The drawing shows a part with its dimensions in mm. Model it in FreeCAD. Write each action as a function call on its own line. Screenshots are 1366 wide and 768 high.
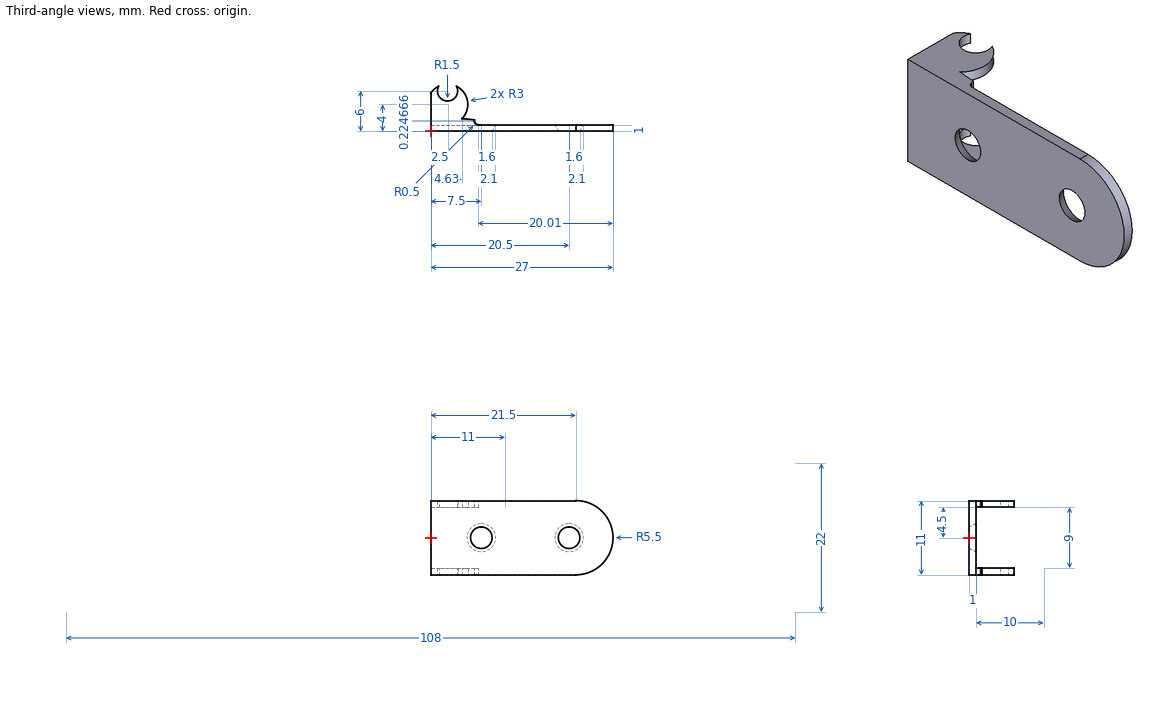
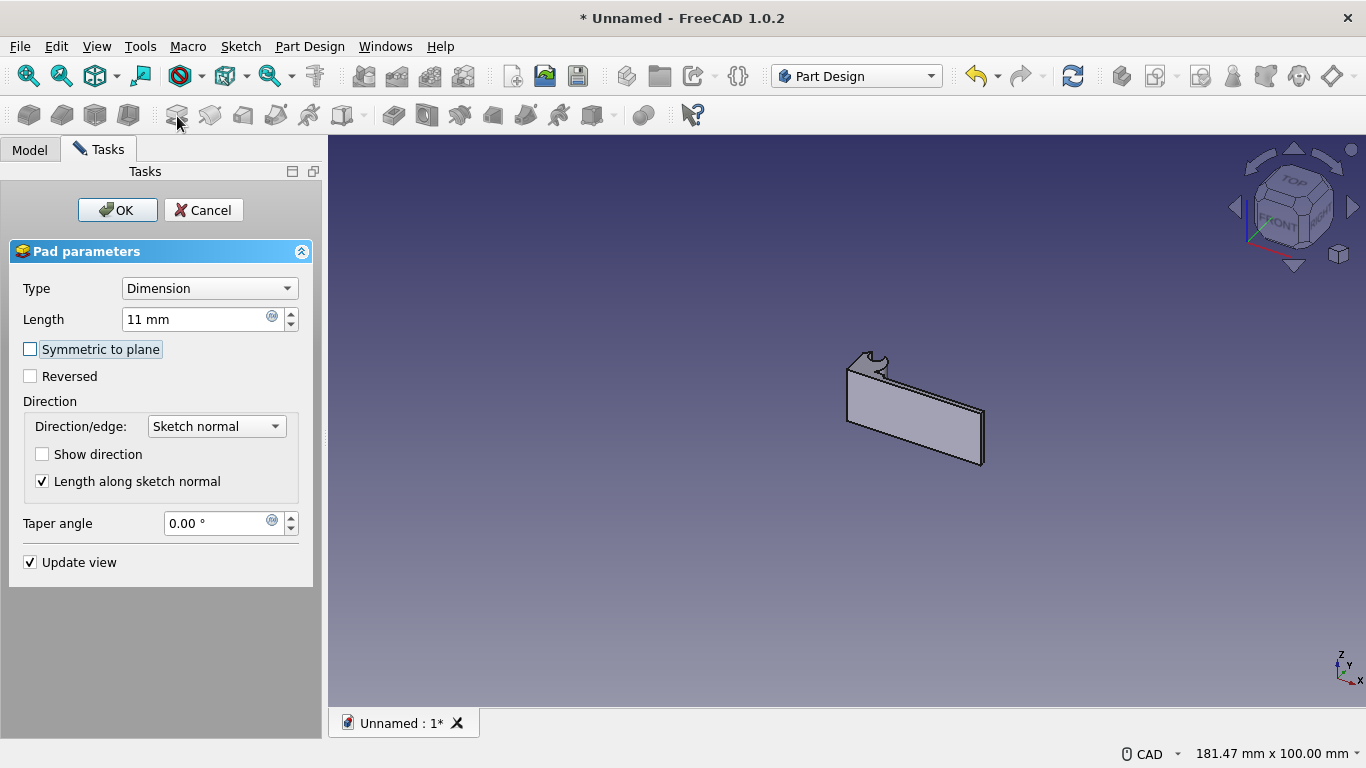
click(31, 349)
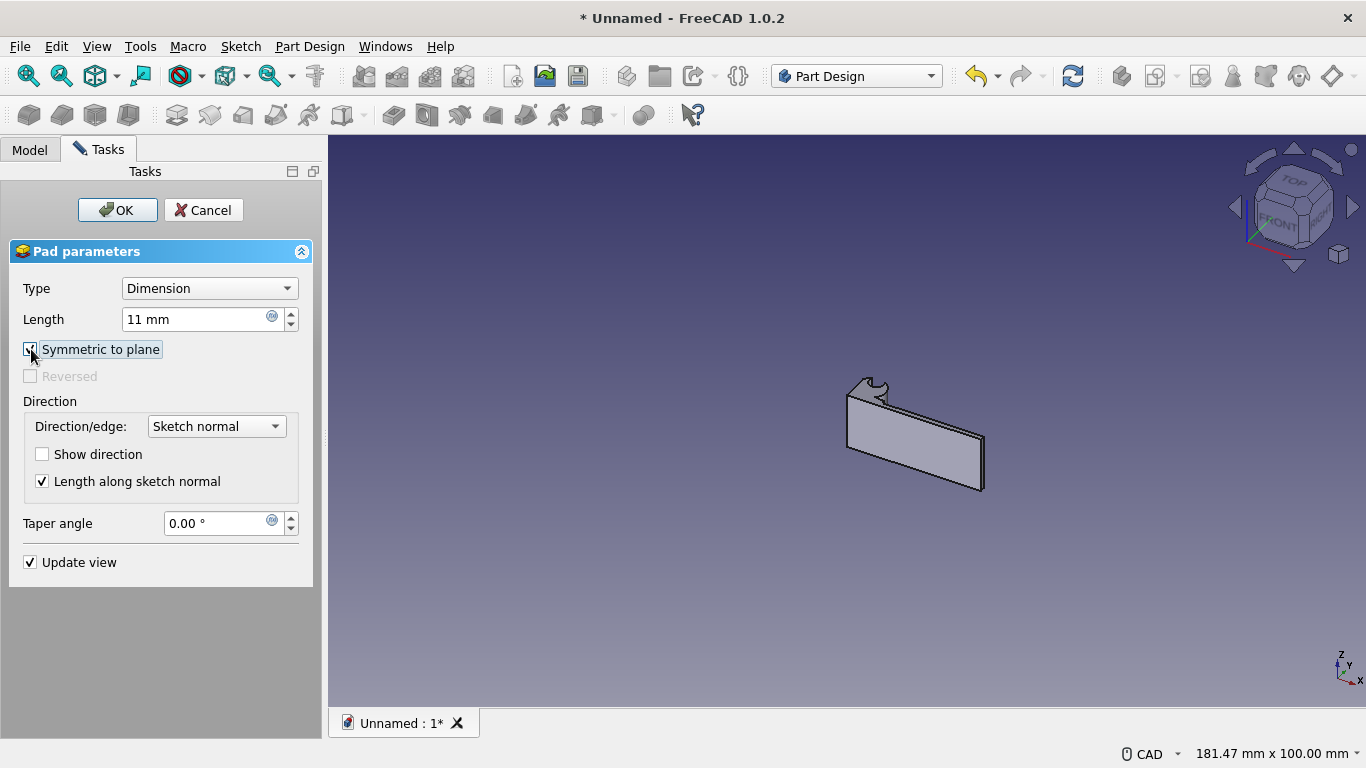
click(118, 210)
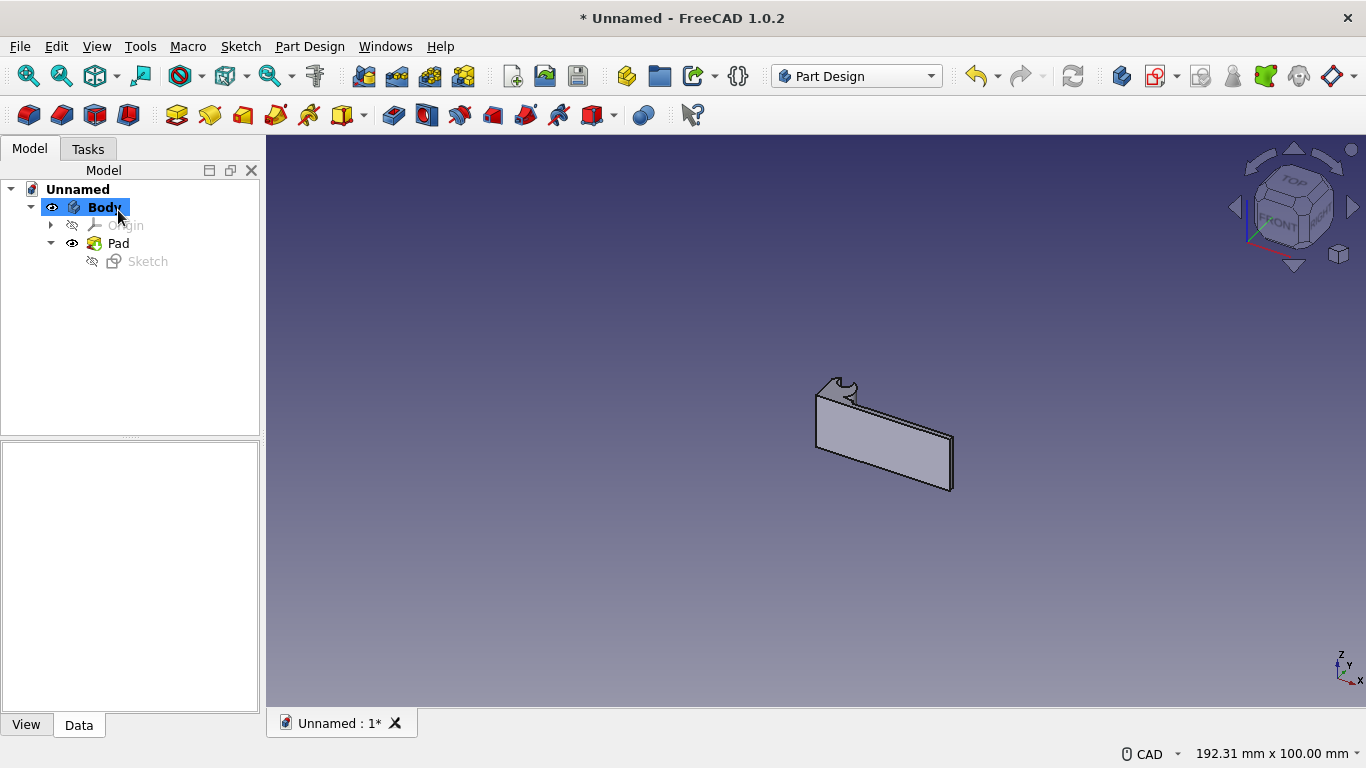
key(v)
key(f)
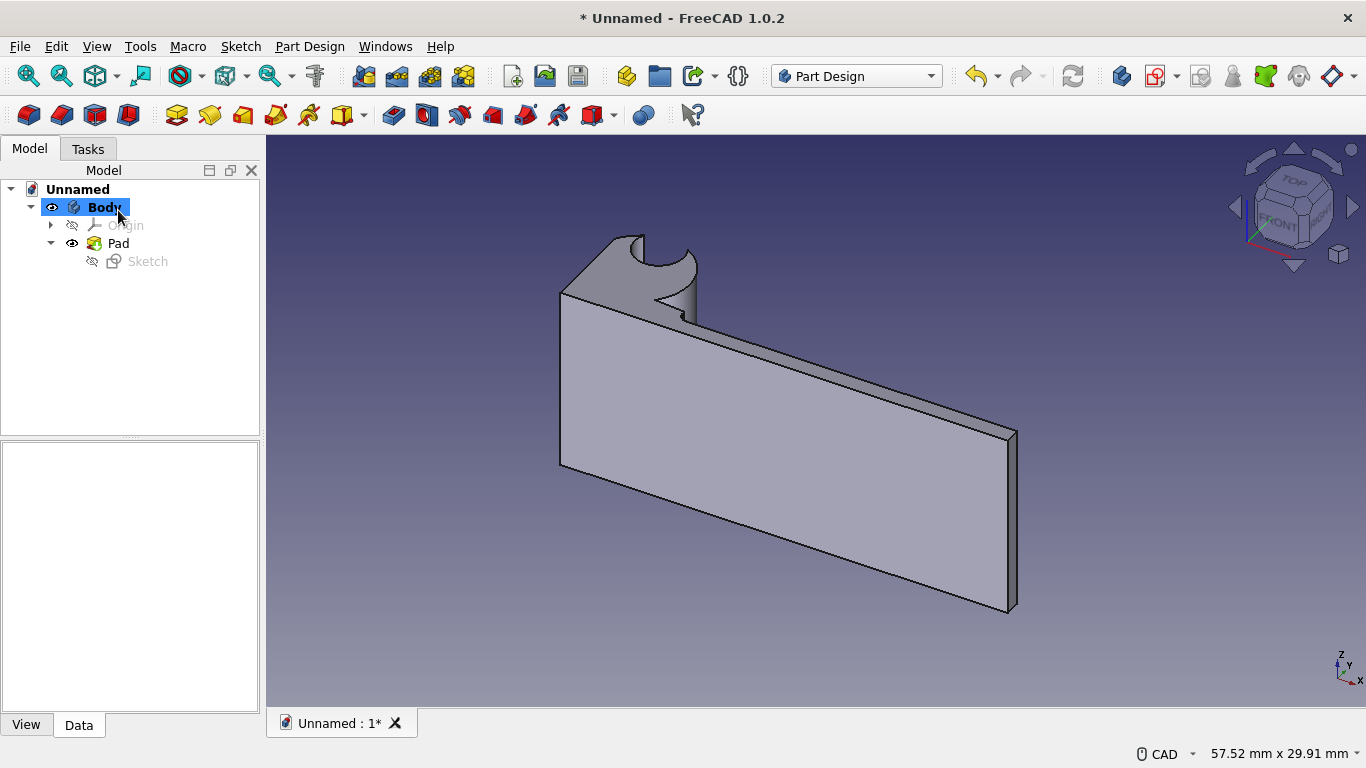
click(1154, 76)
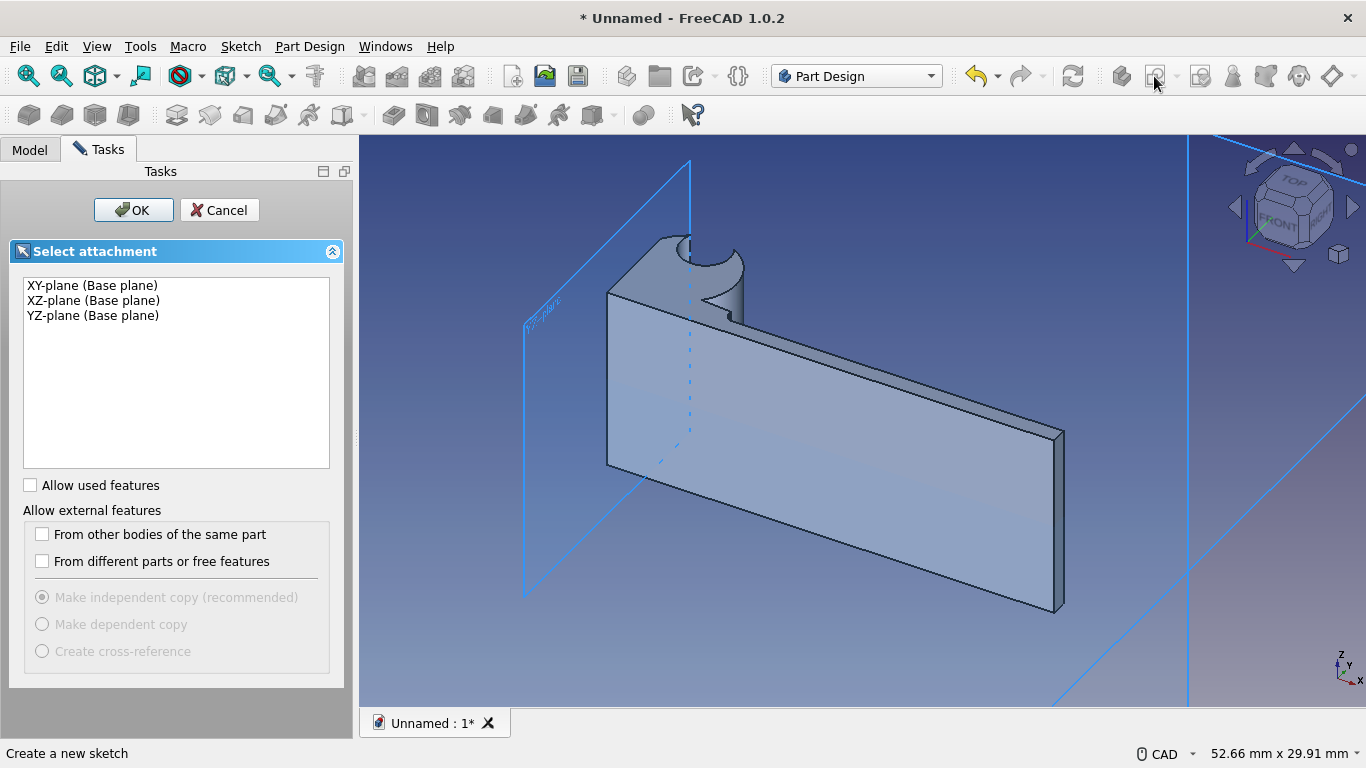
click(84, 300)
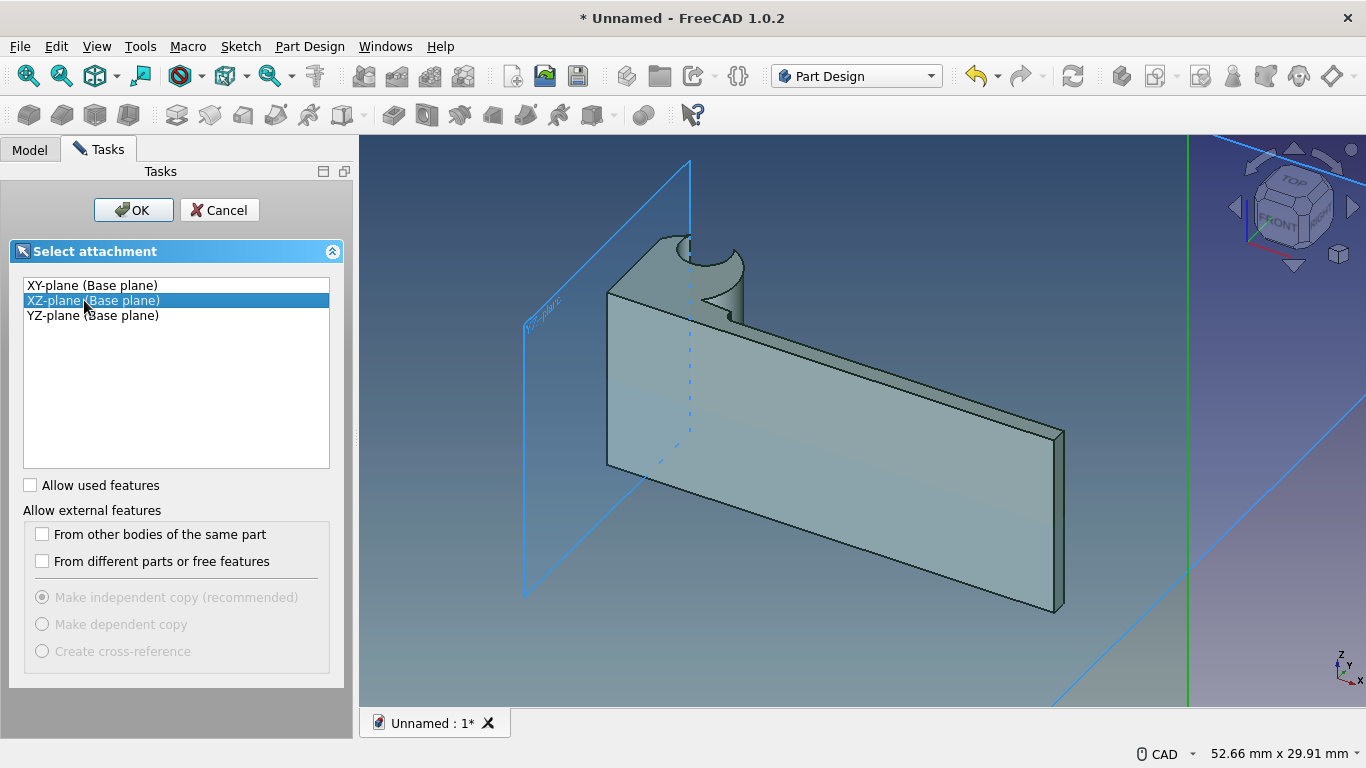
click(134, 210)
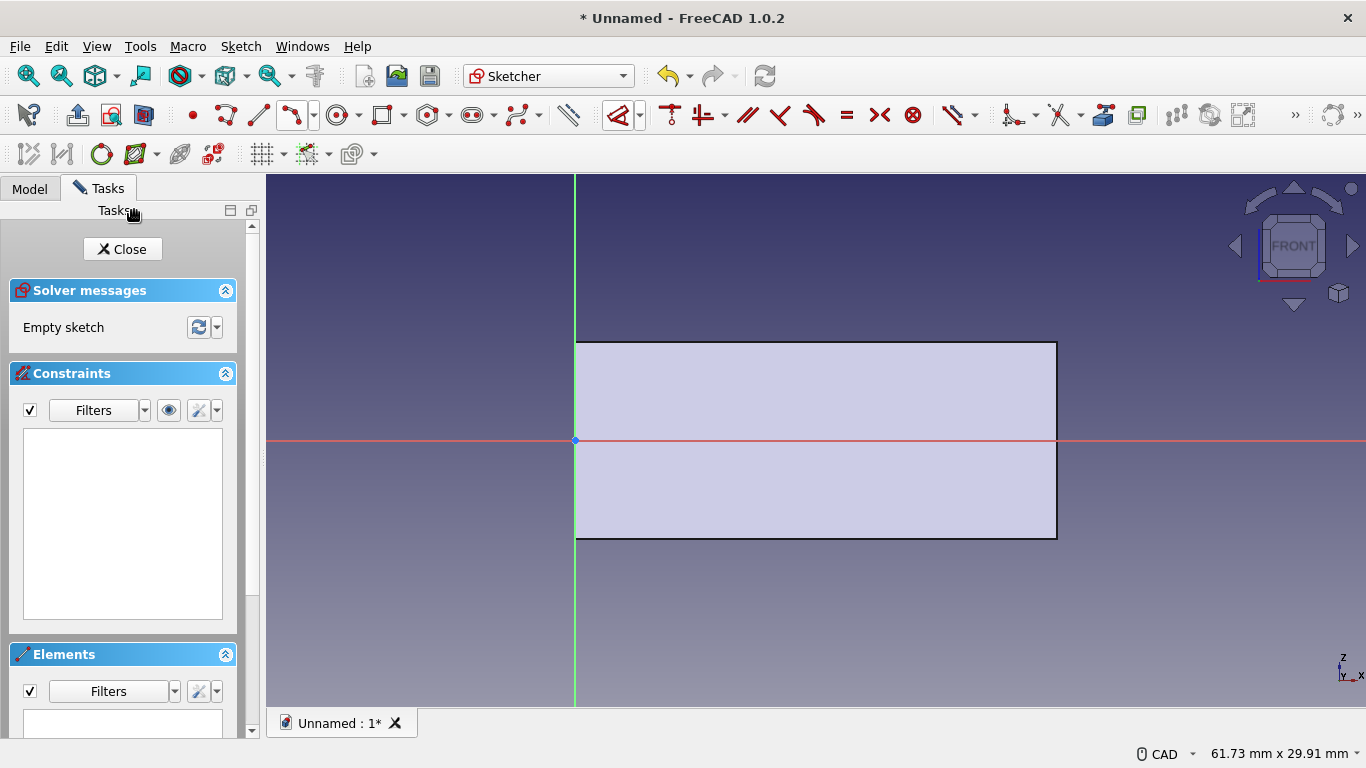
scroll(822, 440, down, 6)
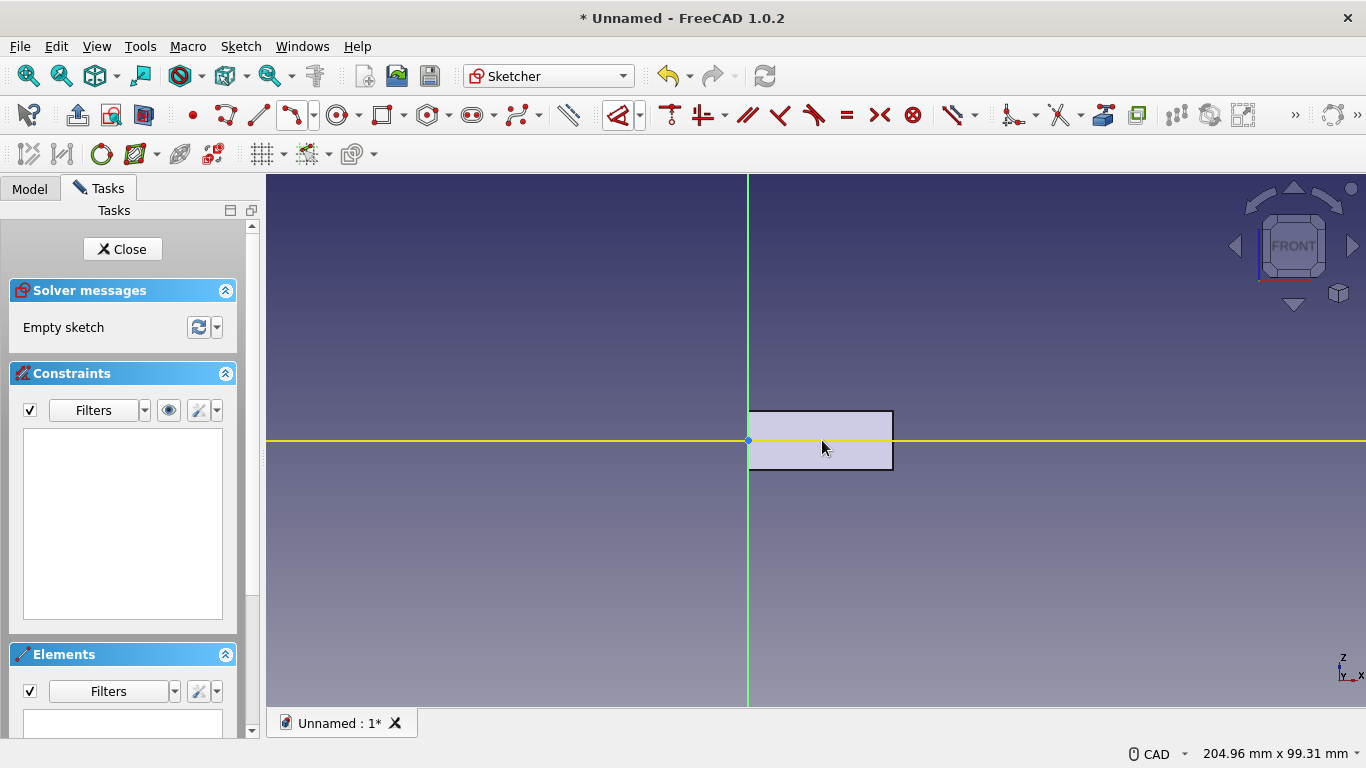
click(404, 116)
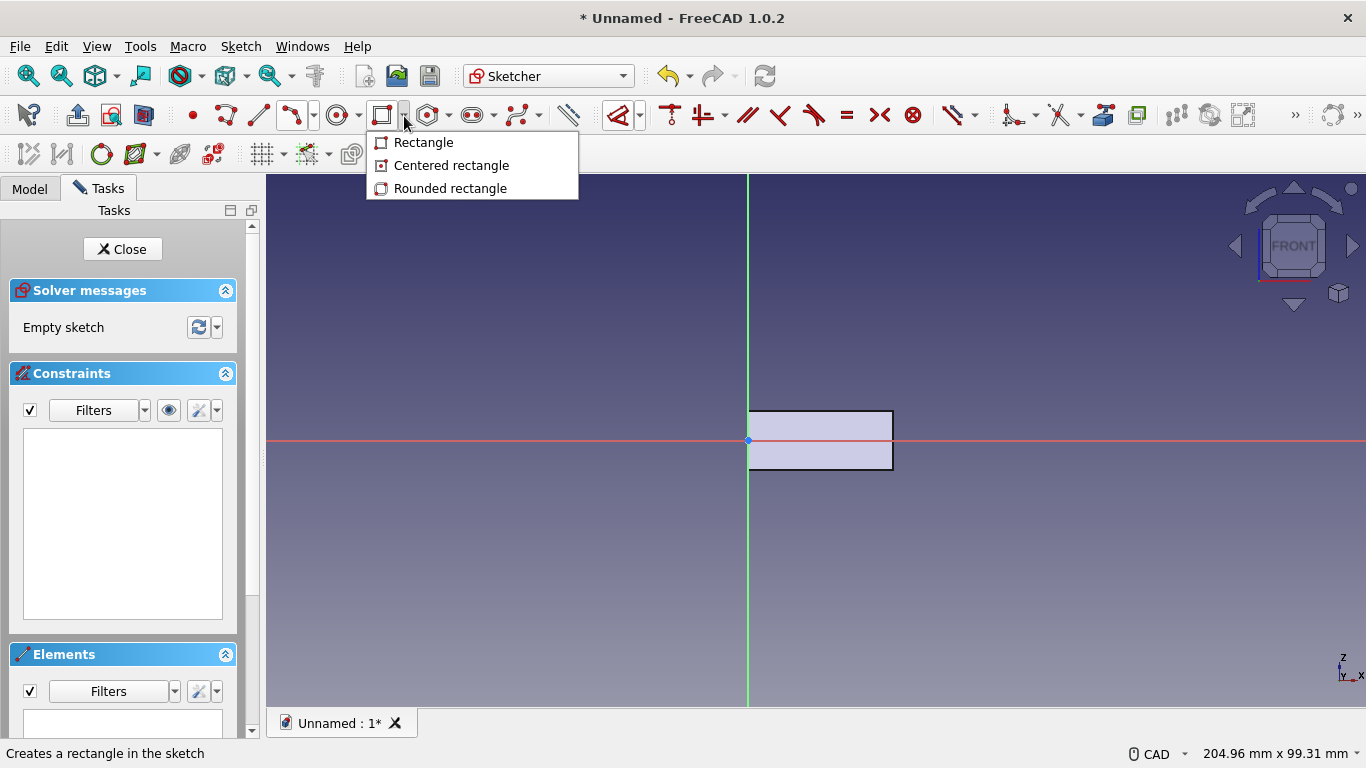
click(472, 166)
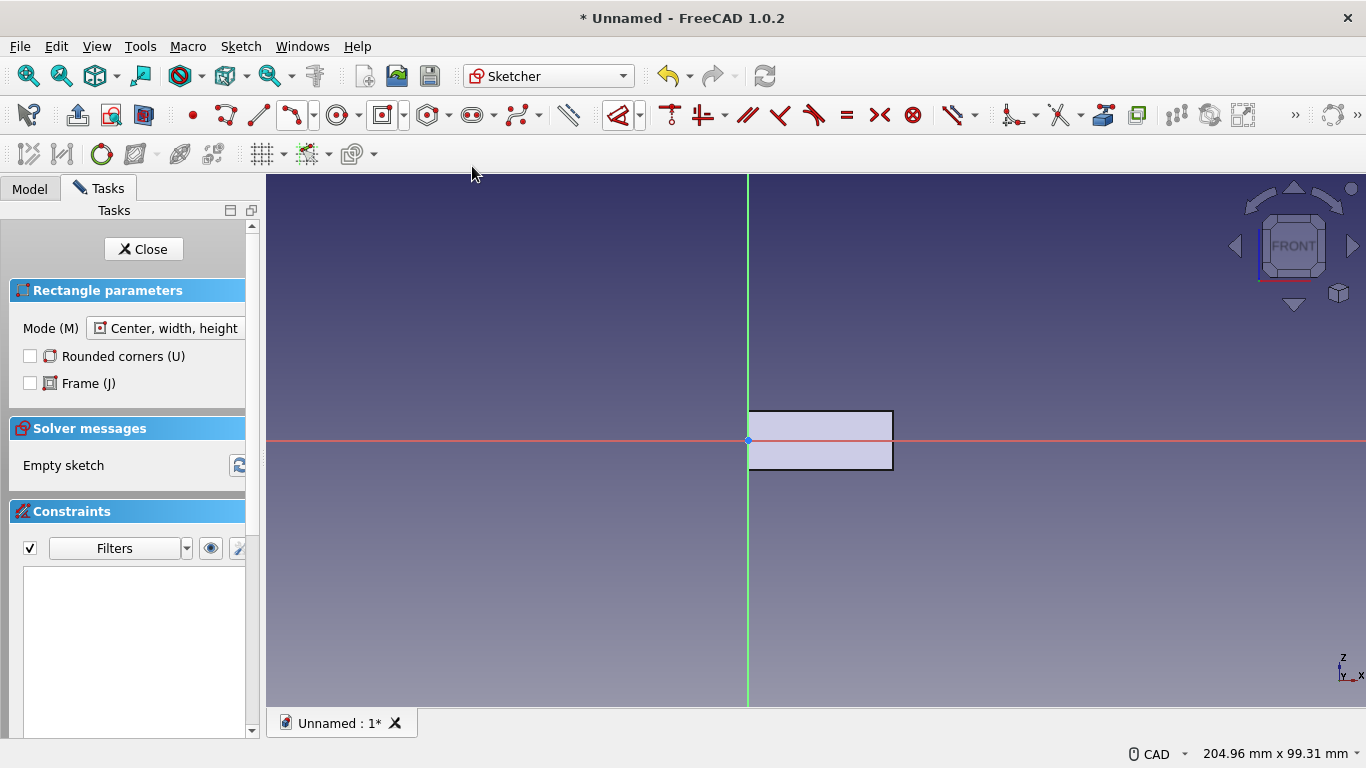
click(748, 441)
click(1038, 381)